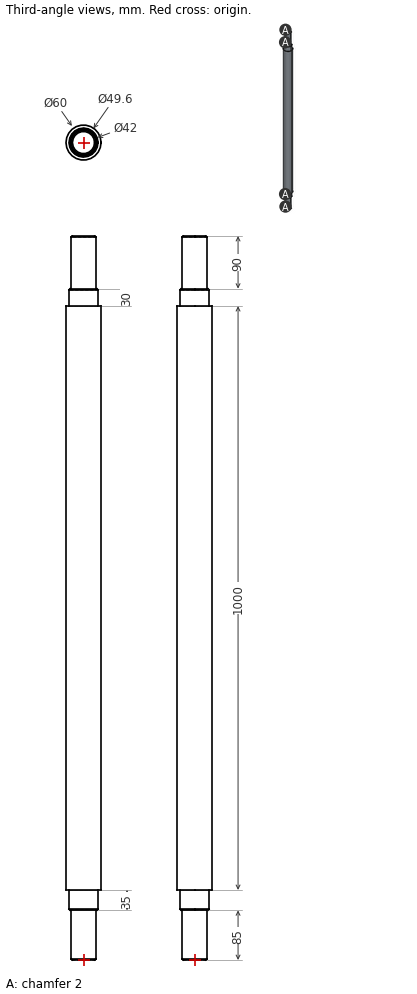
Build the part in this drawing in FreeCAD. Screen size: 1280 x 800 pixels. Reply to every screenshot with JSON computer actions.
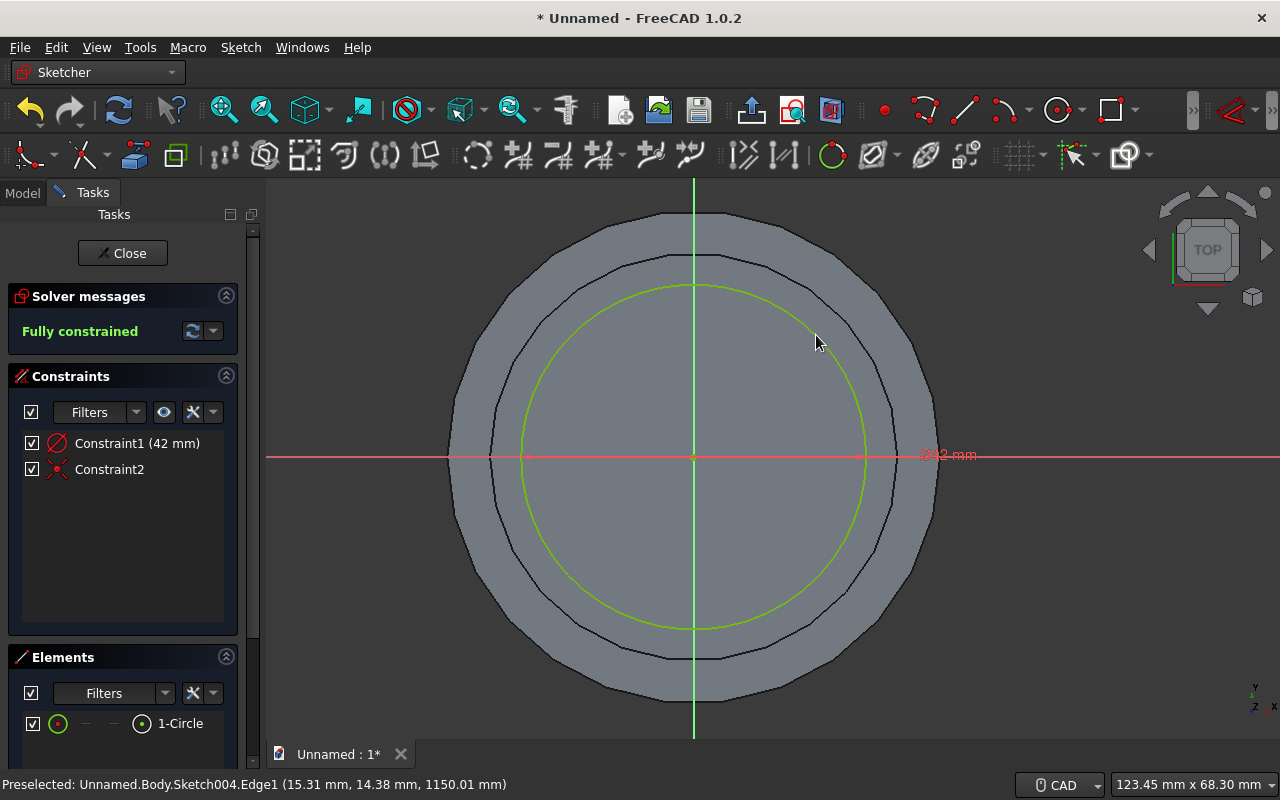
{"action": "left_click", "coordinate": [123, 253]}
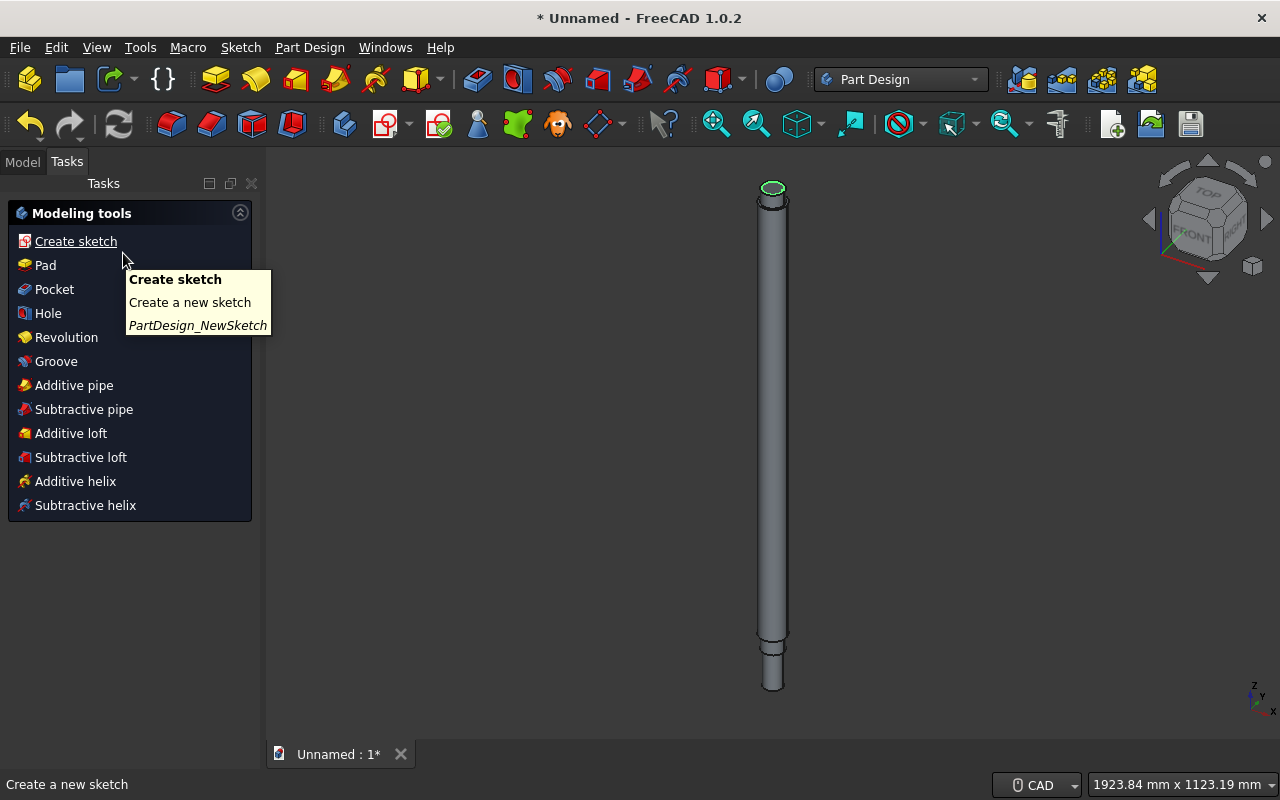
{"action": "left_click", "coordinate": [216, 80]}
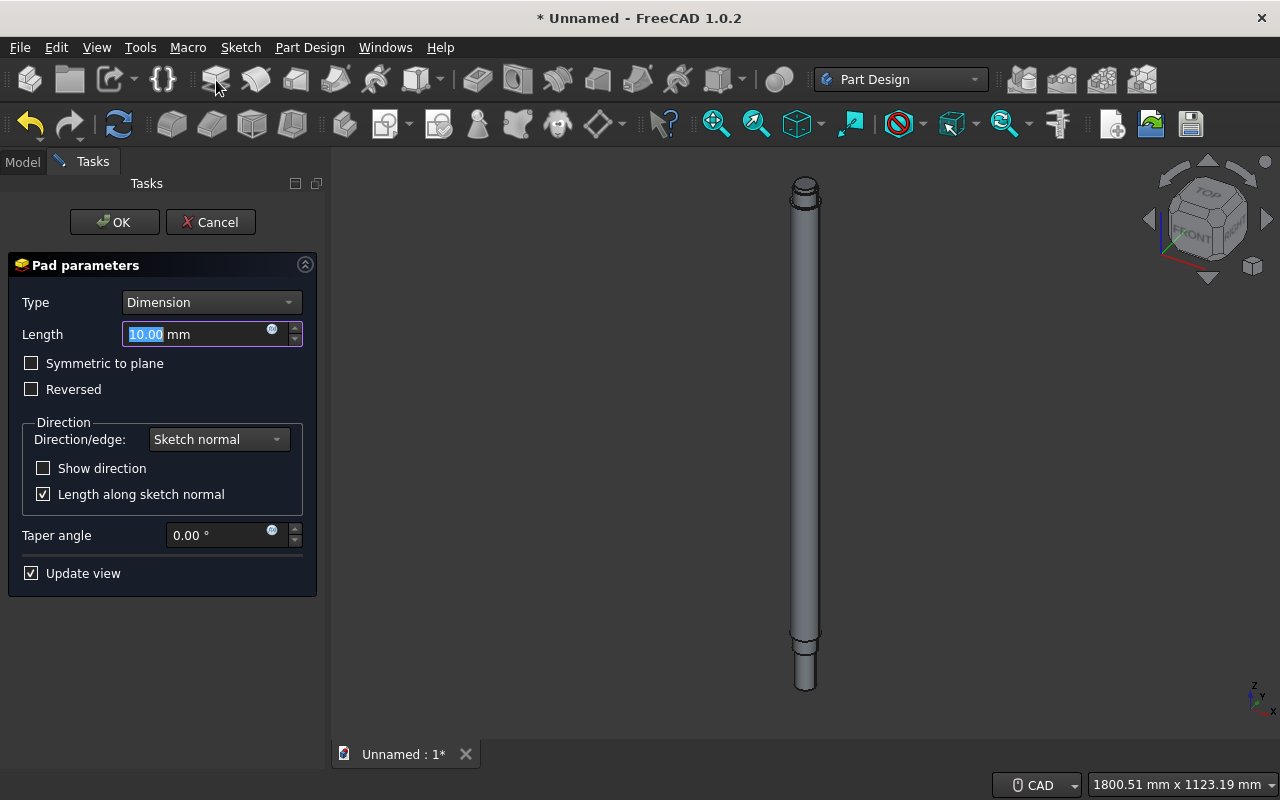
{"action": "type", "text": "90"}
{"action": "key", "text": "Tab"}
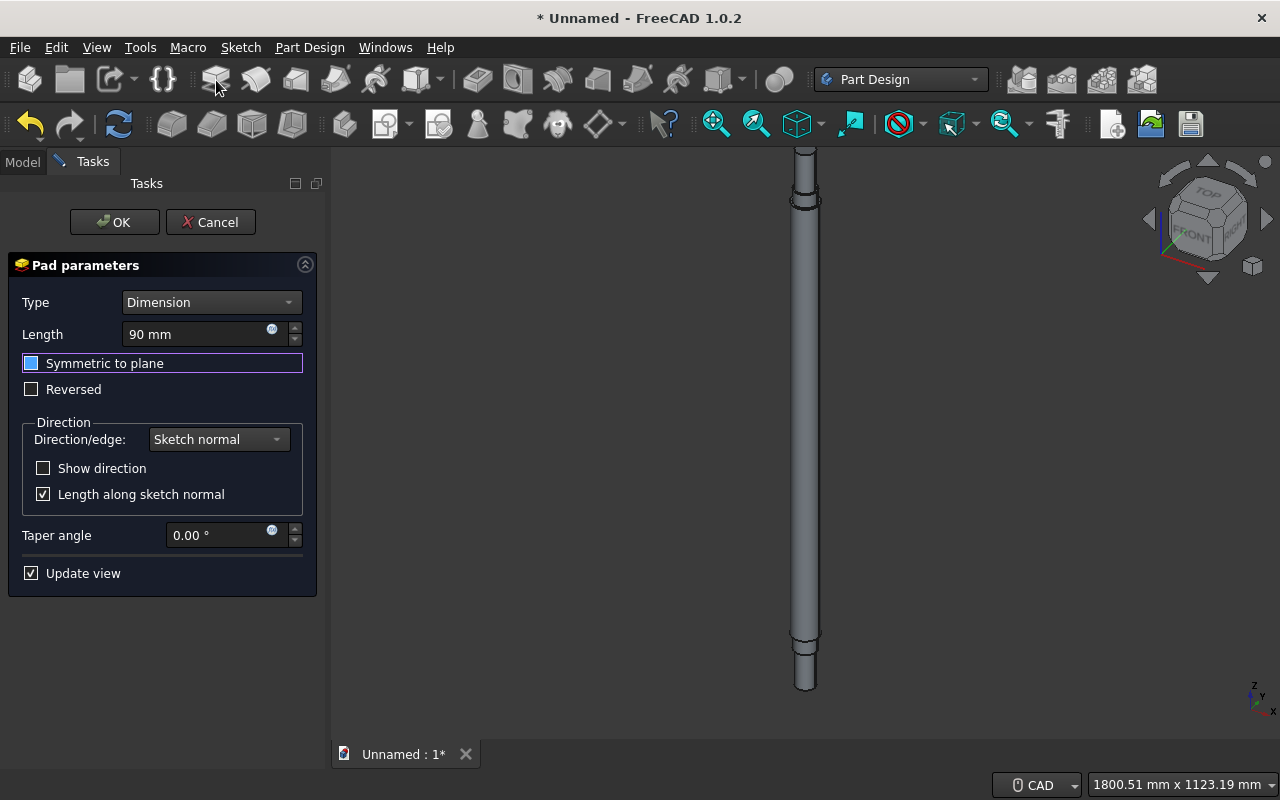
{"action": "left_click", "coordinate": [115, 222]}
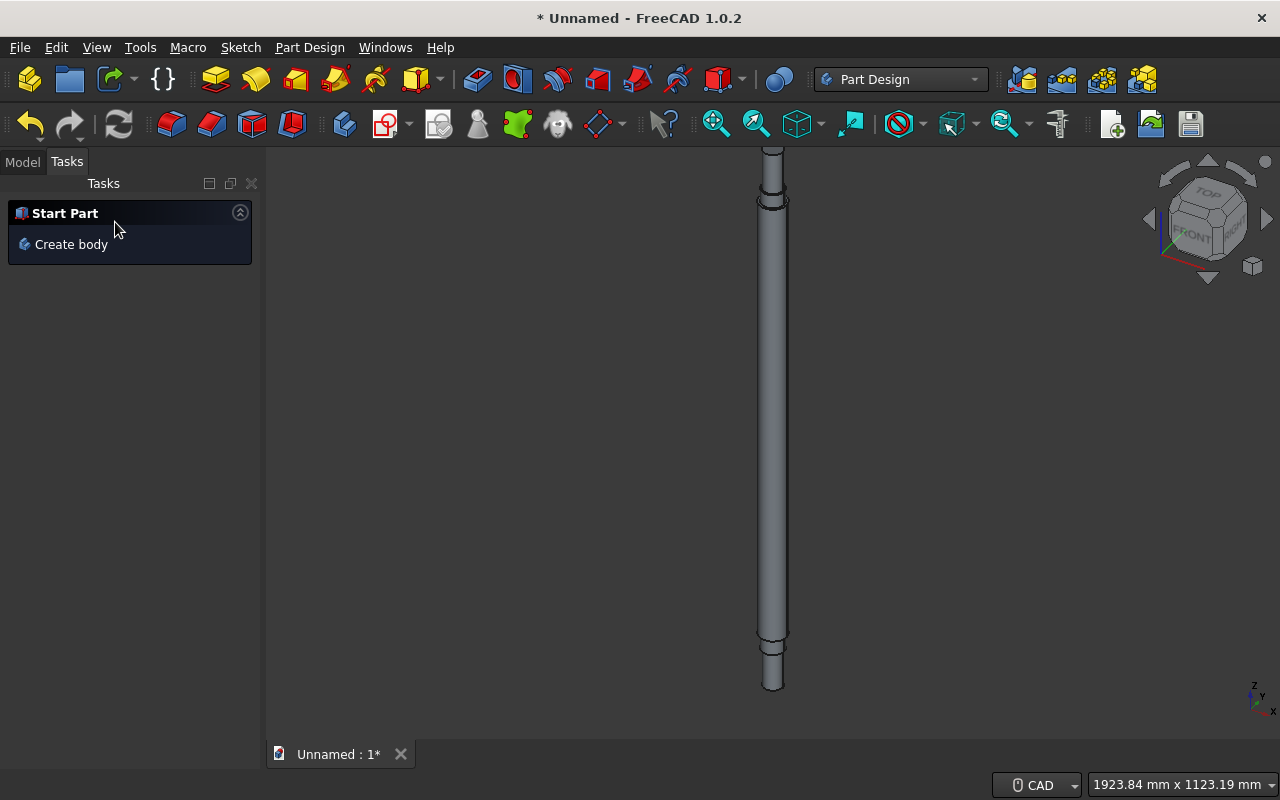
{"action": "left_click", "coordinate": [718, 124]}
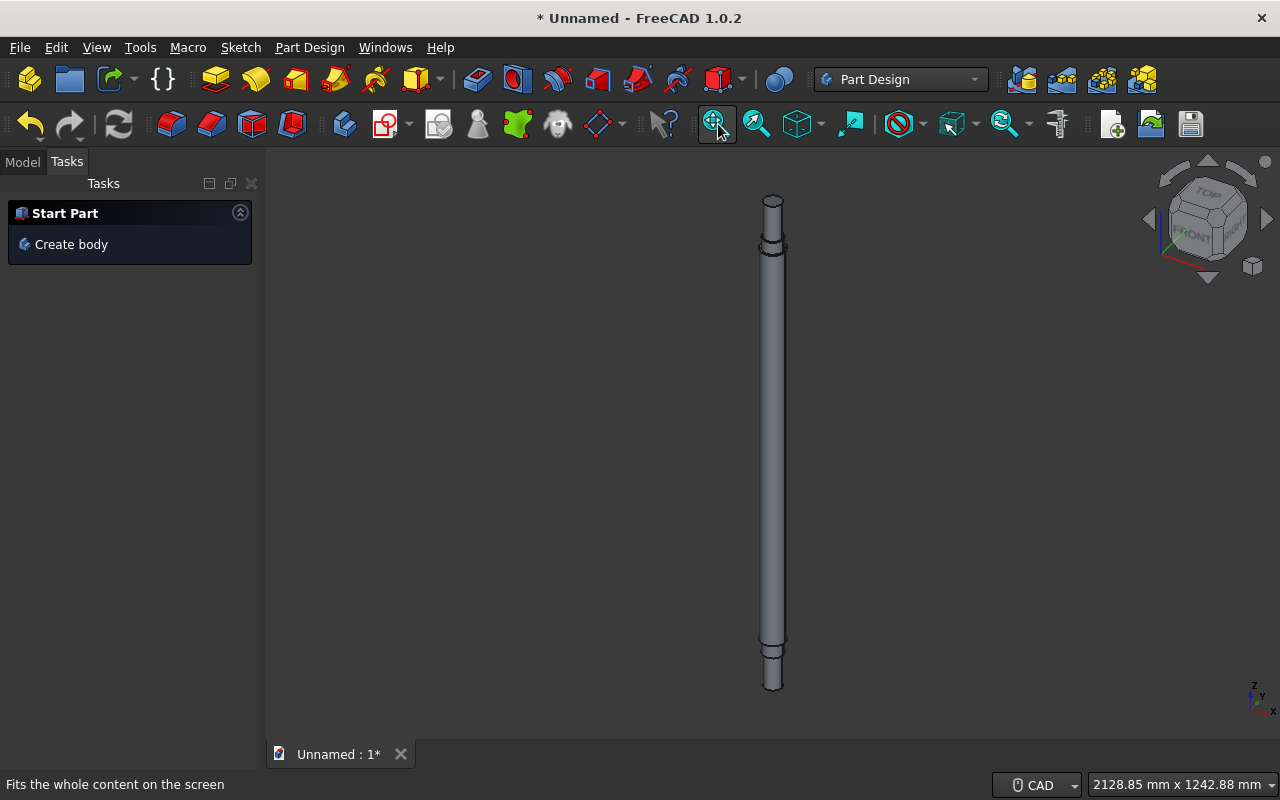
{"action": "left_click", "coordinate": [761, 236]}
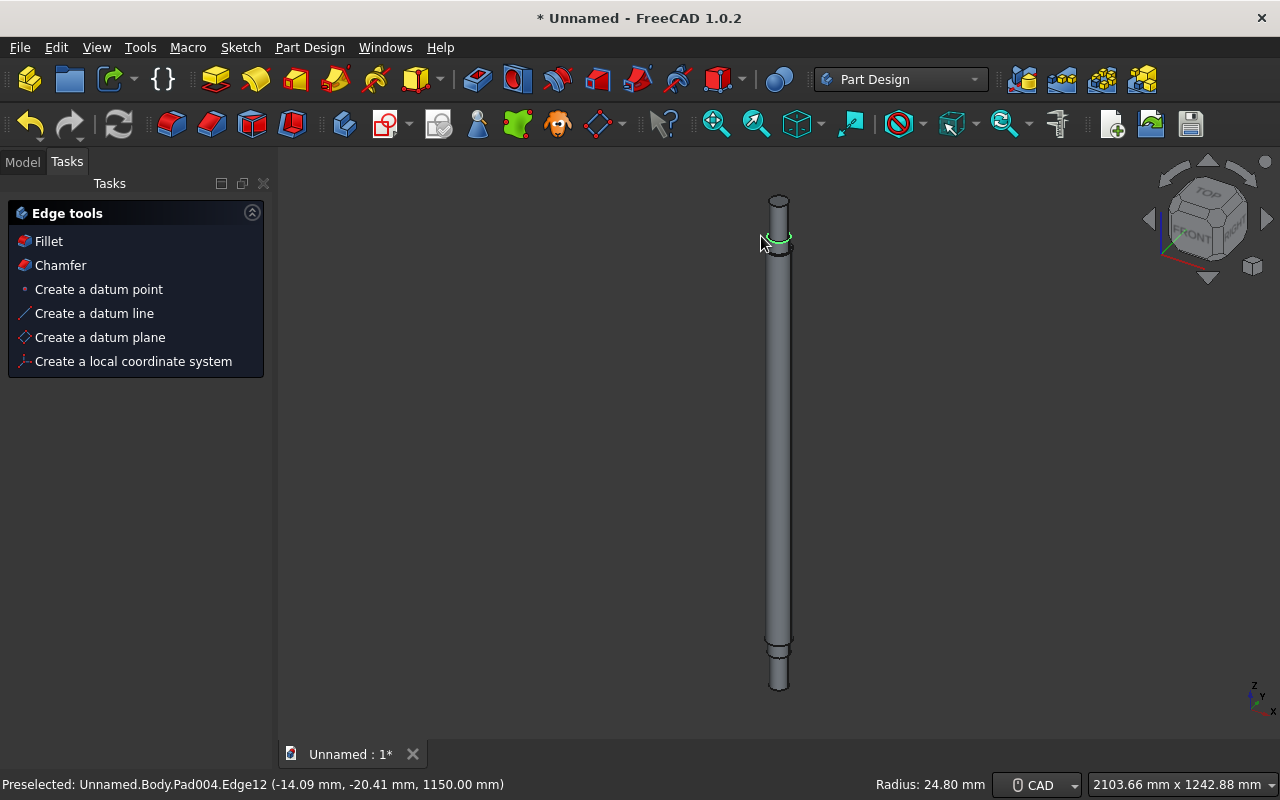
{"action": "left_click", "coordinate": [770, 197], "text": "ctrl"}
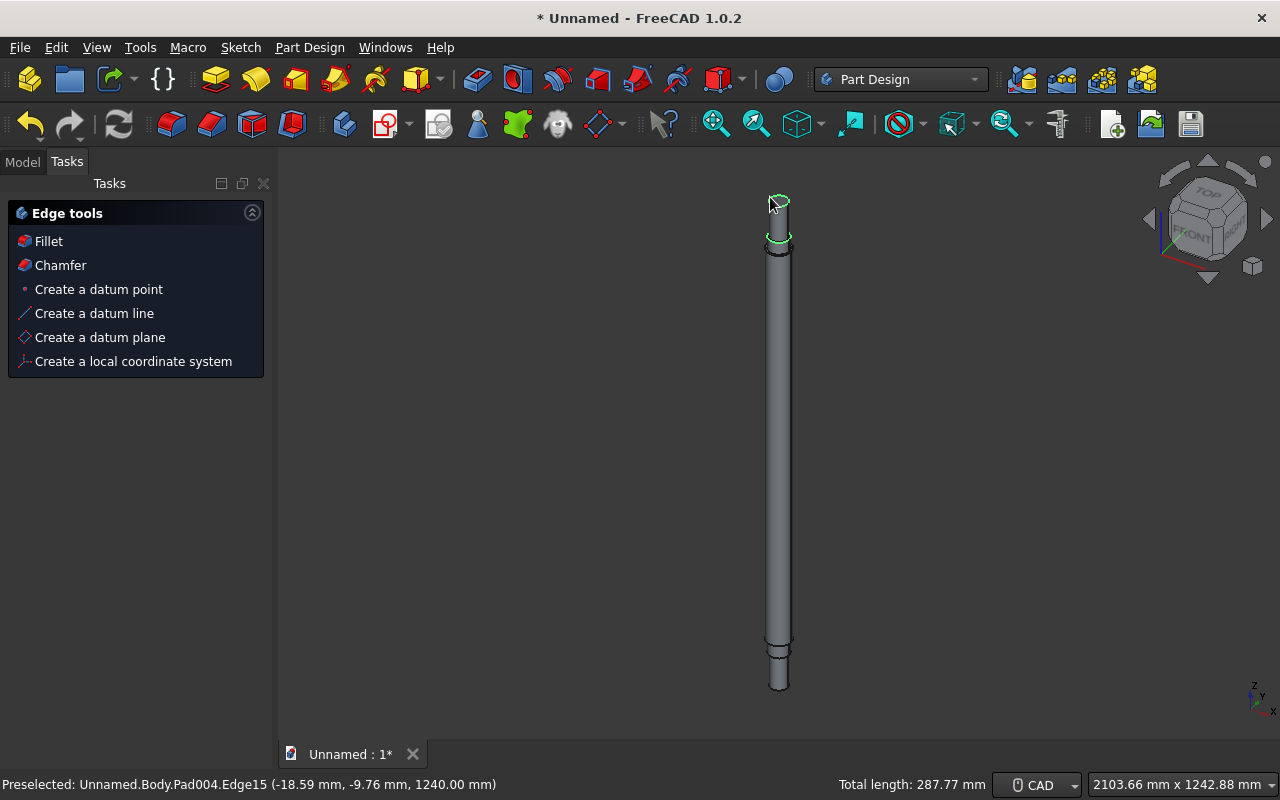
{"action": "left_click", "coordinate": [788, 686], "text": "ctrl"}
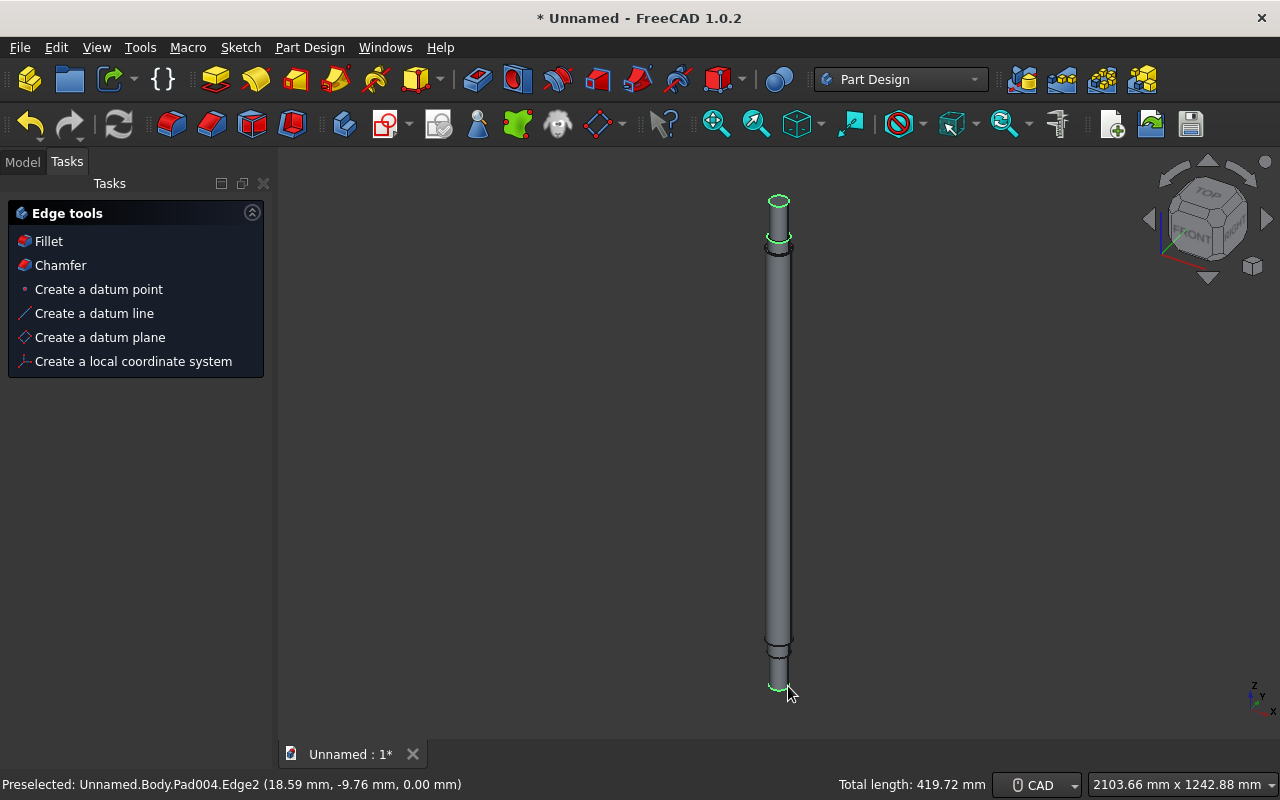
{"action": "left_click", "coordinate": [770, 655], "text": "ctrl"}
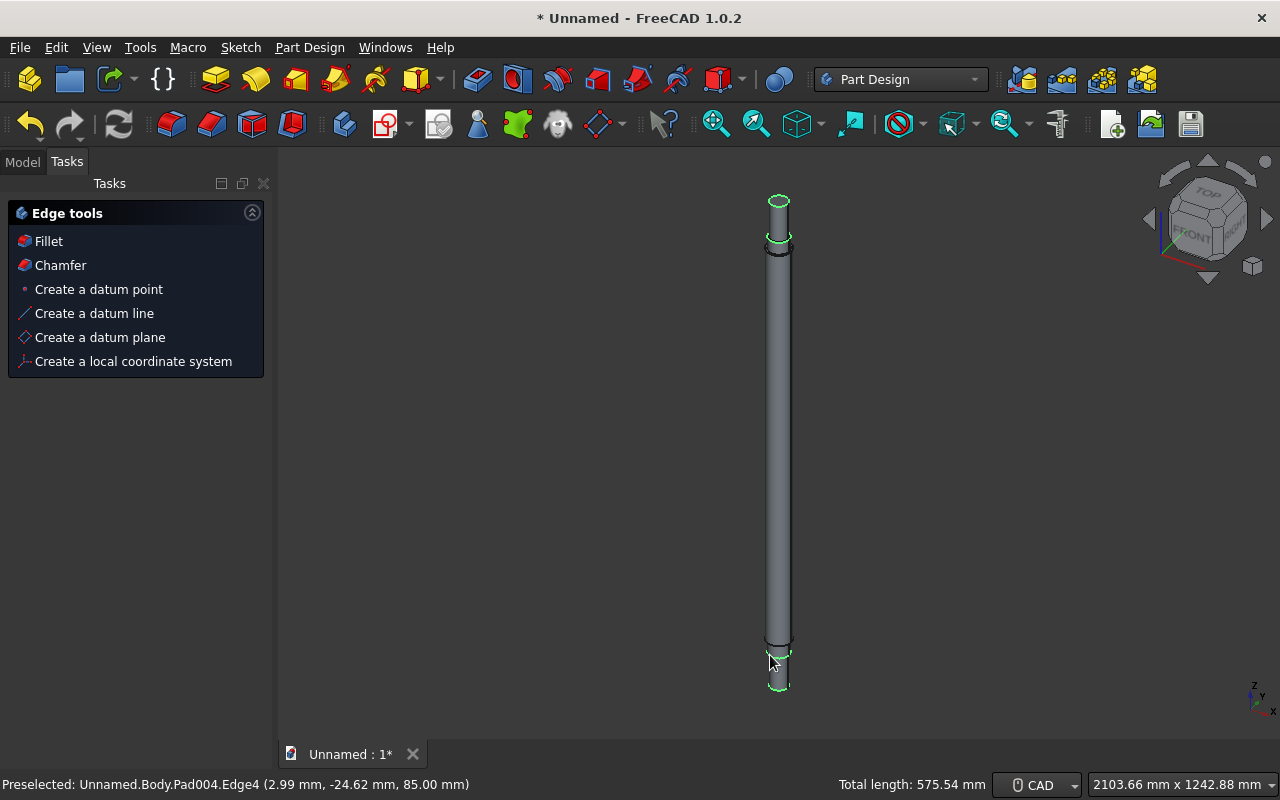
{"action": "left_click", "coordinate": [212, 124]}